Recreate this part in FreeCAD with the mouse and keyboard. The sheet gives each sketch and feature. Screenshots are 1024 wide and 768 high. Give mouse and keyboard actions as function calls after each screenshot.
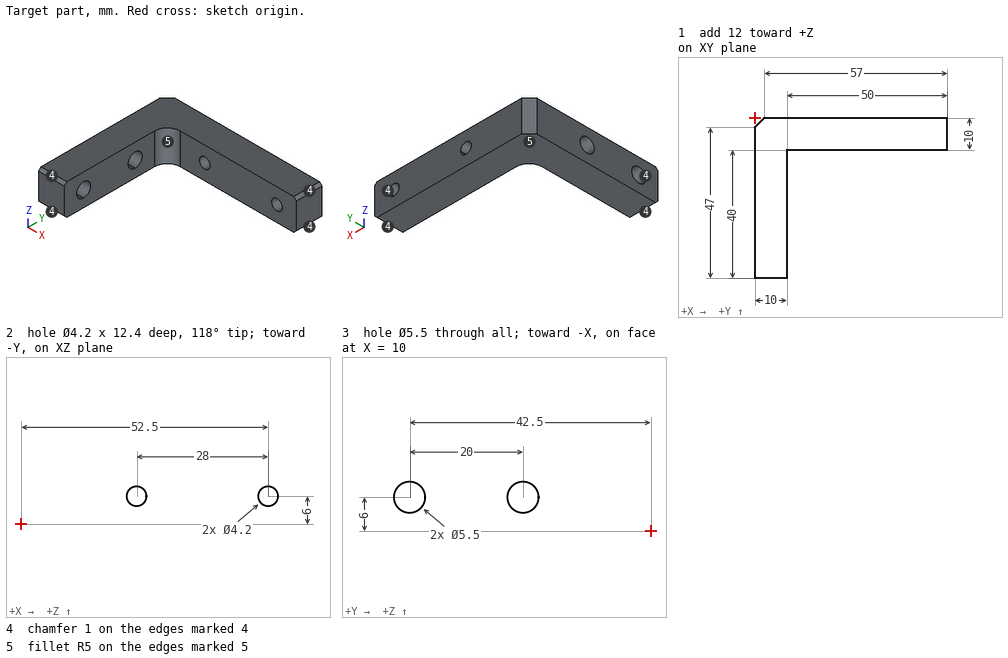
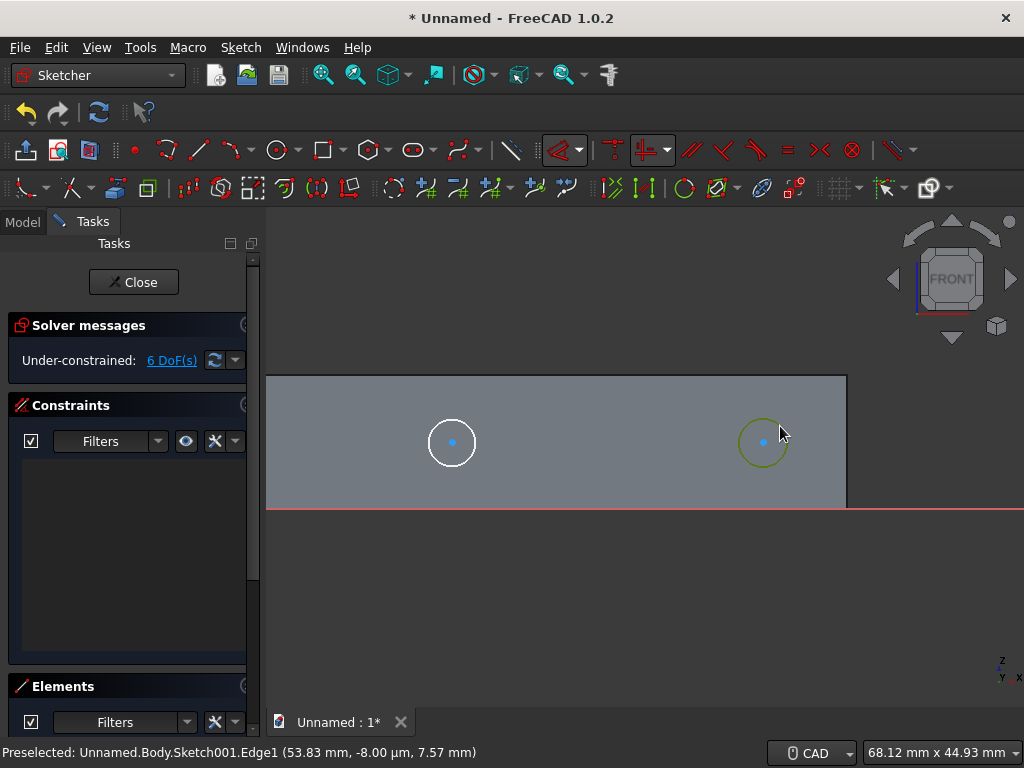
click(468, 426)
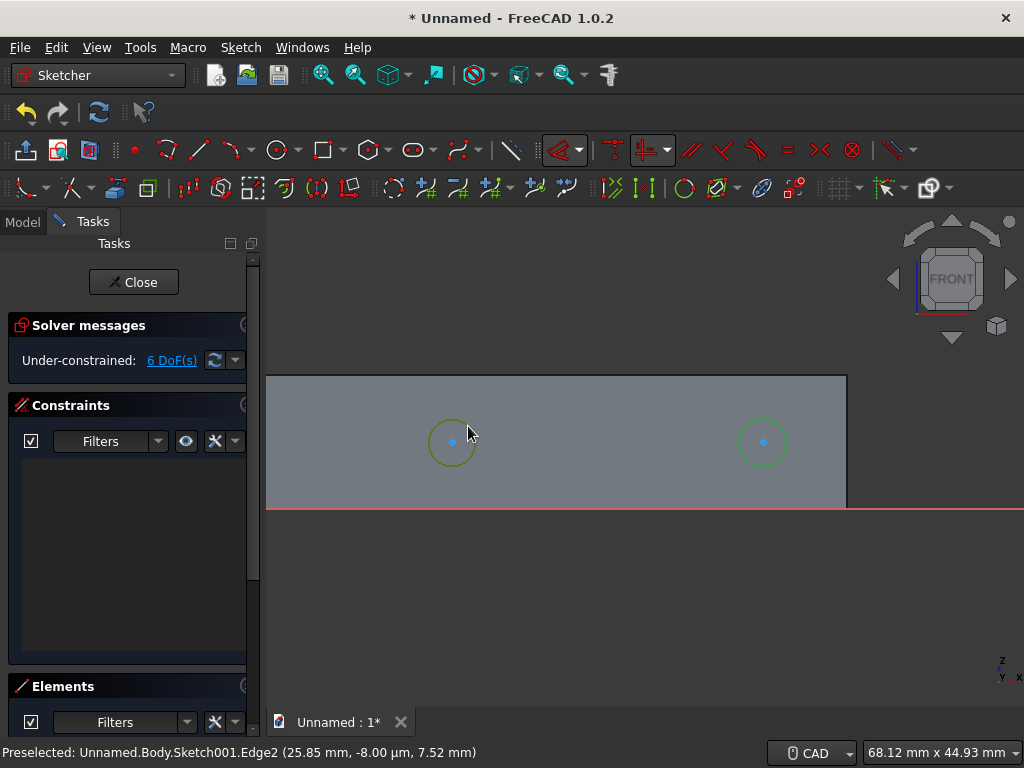
key(e)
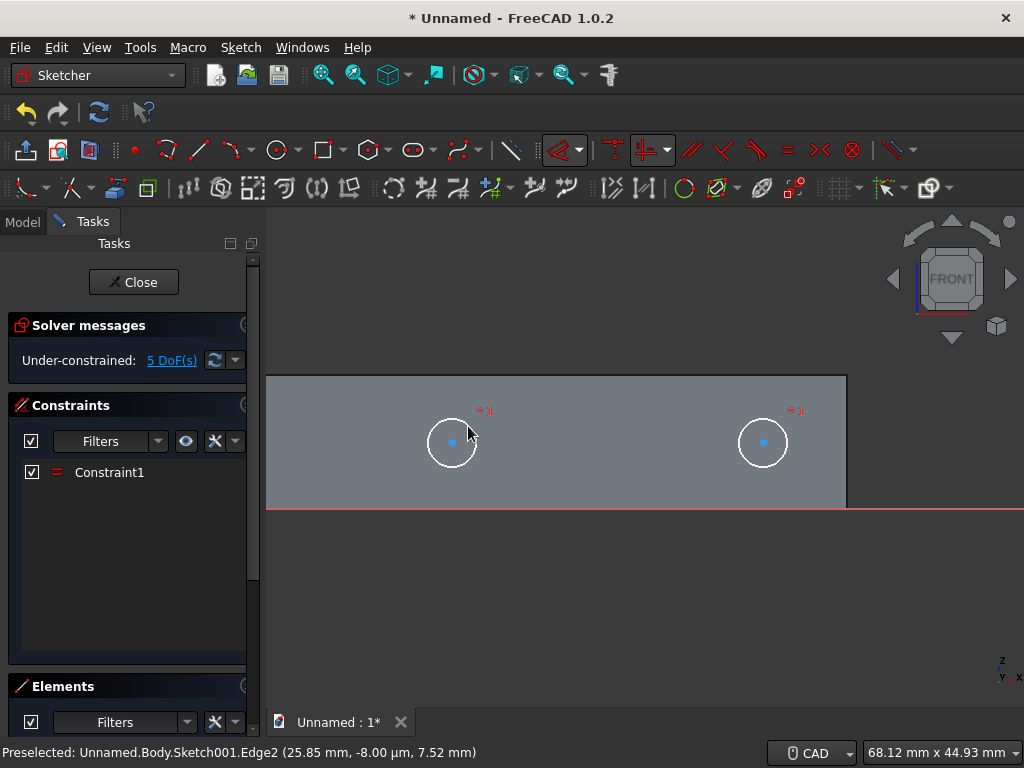
click(763, 443)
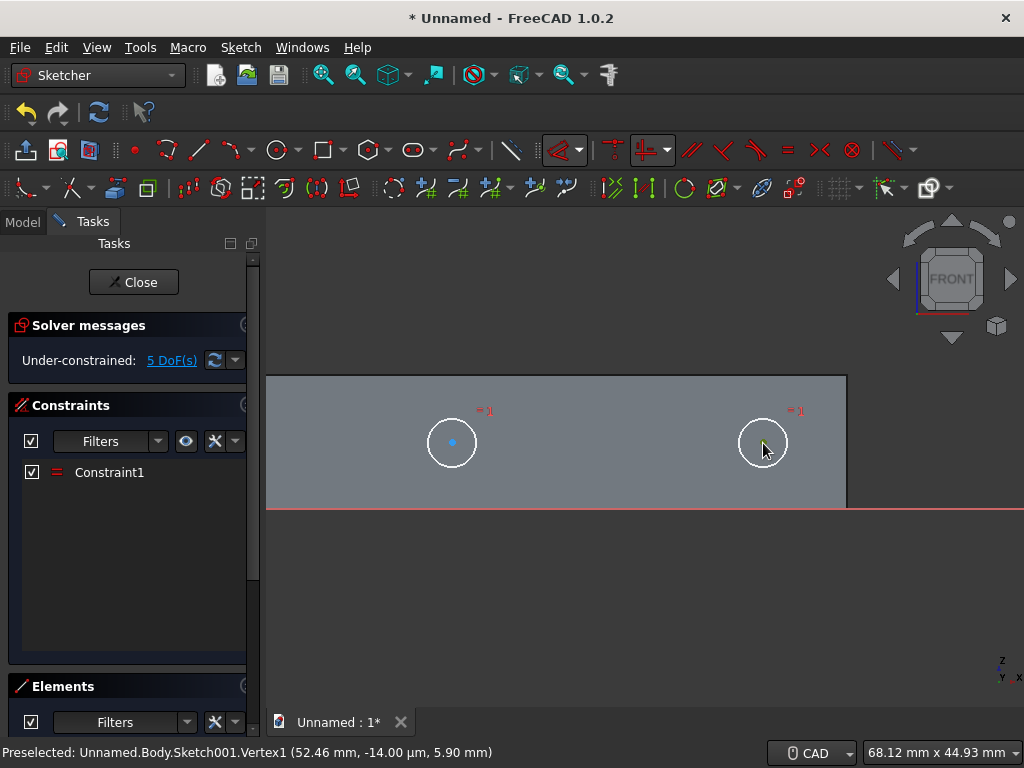
click(452, 443)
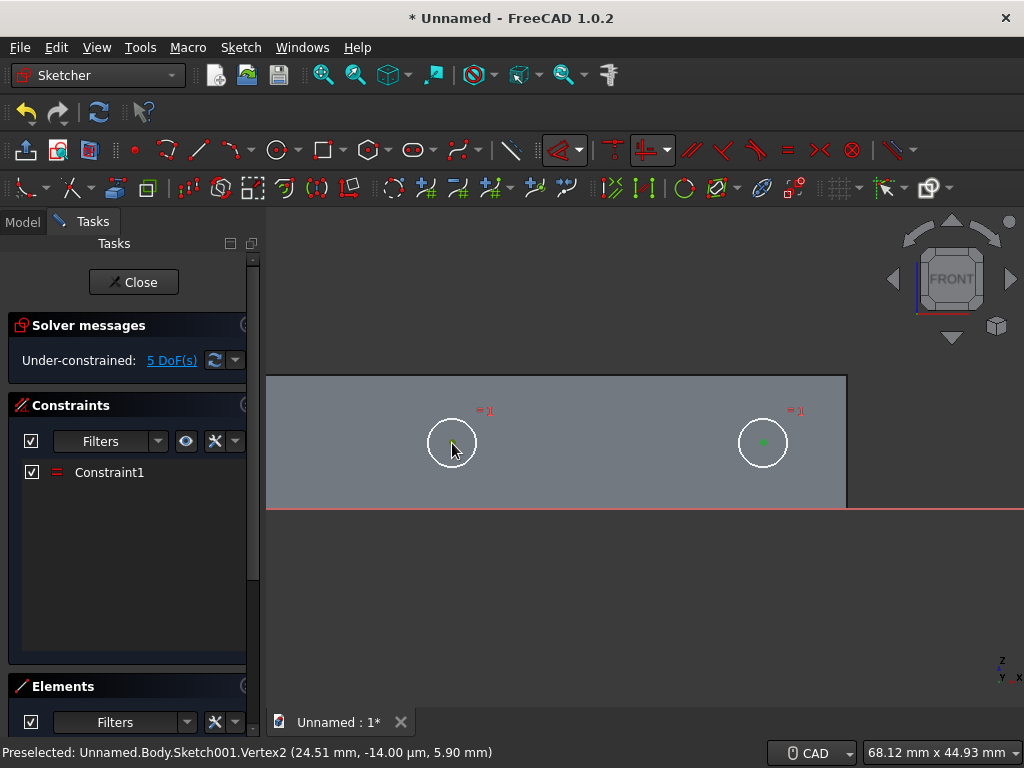
key(h)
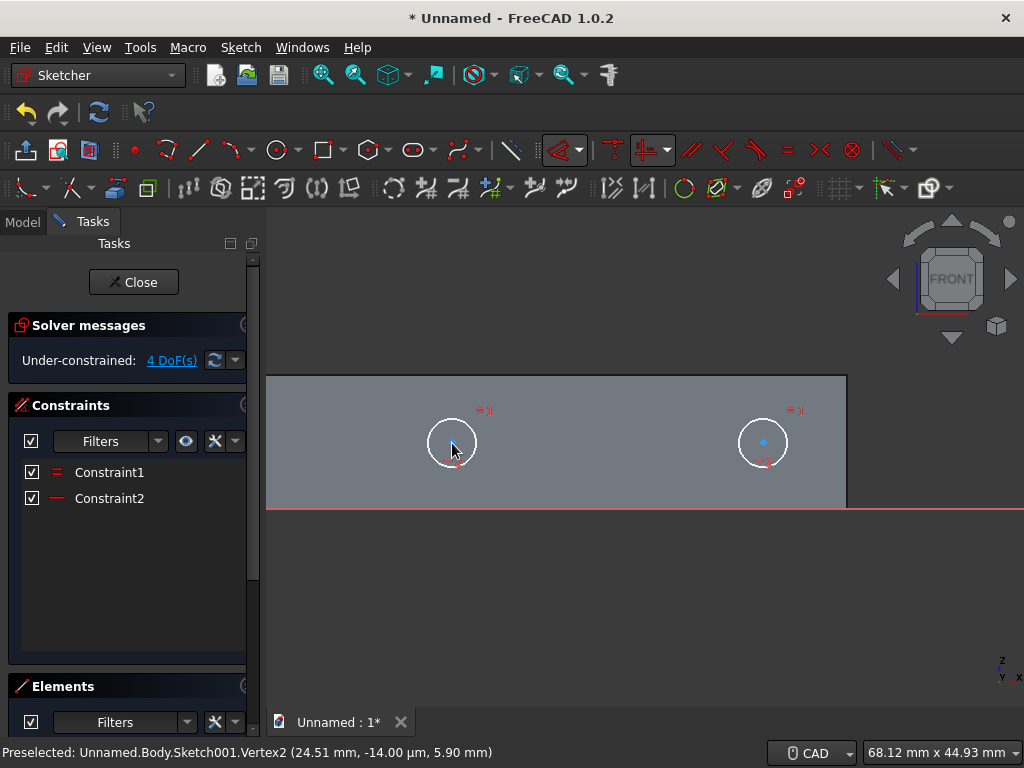
key(d)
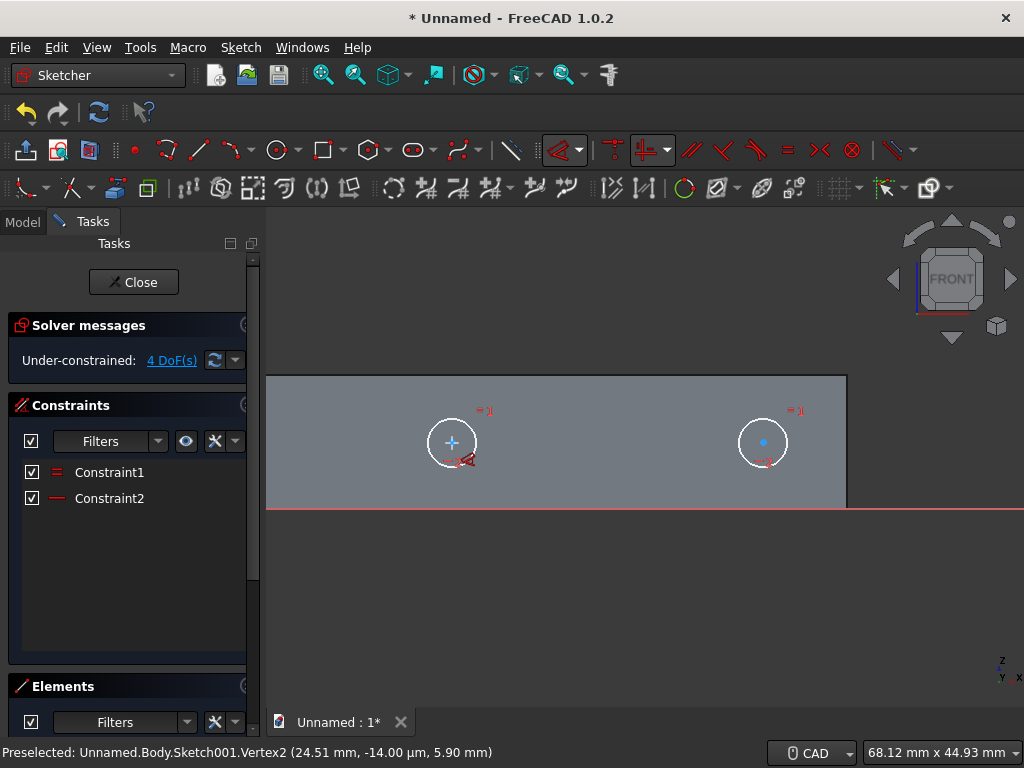
click(780, 426)
click(803, 403)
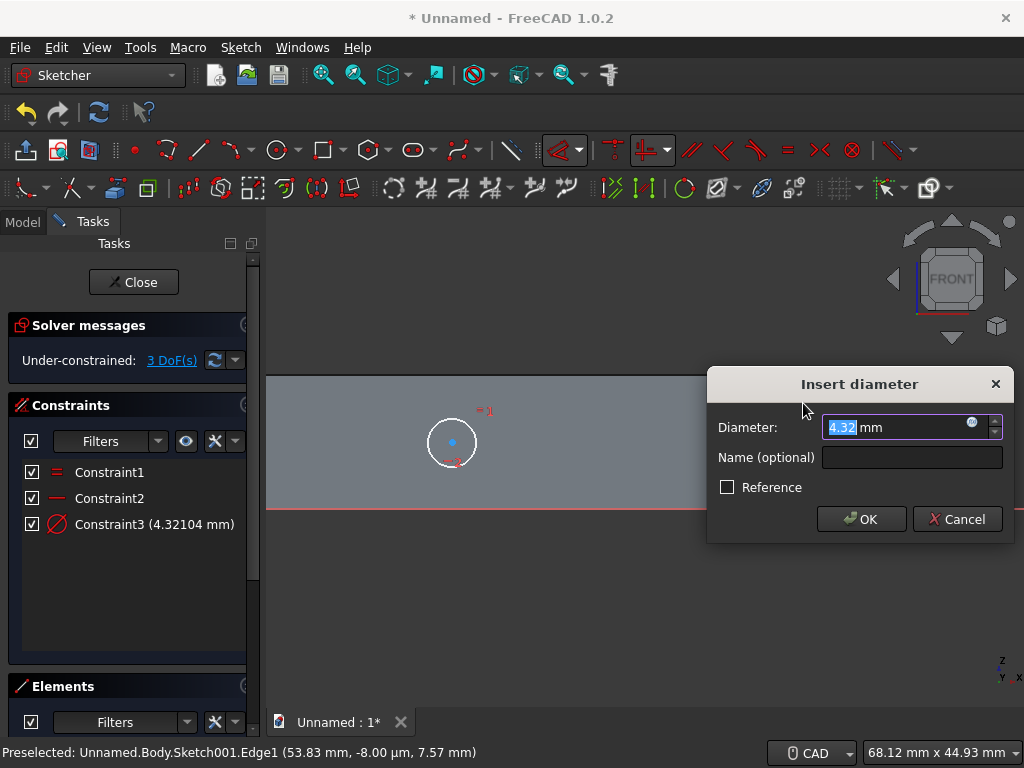
text(4.2)
key(Return)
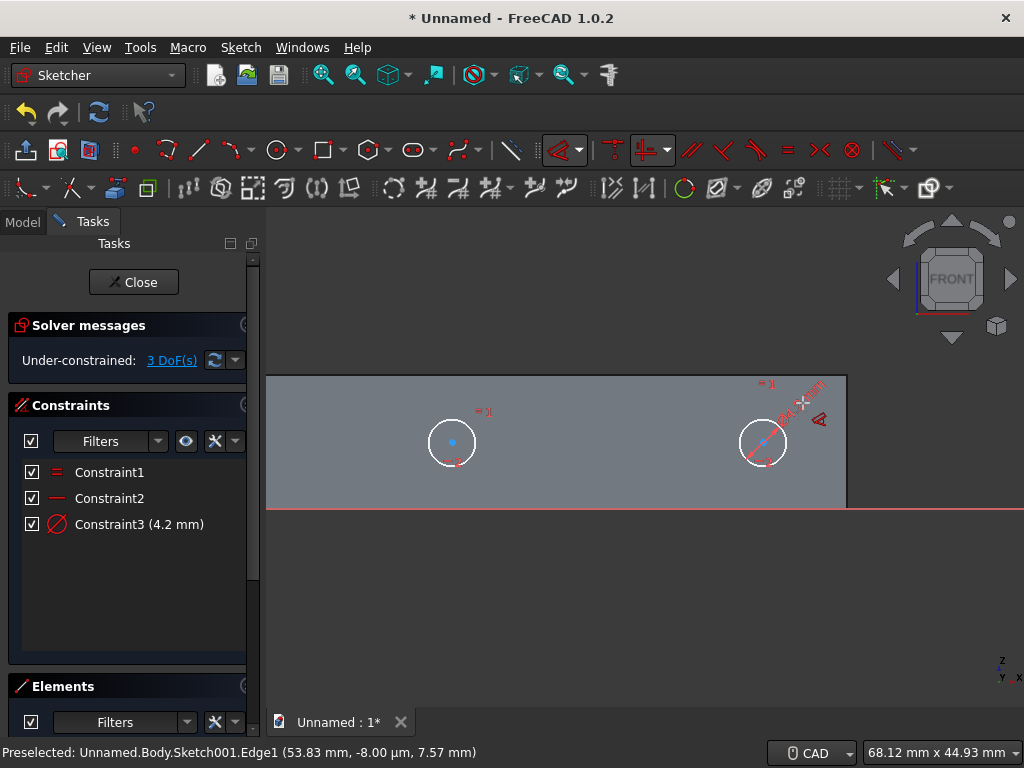
click(763, 443)
click(797, 476)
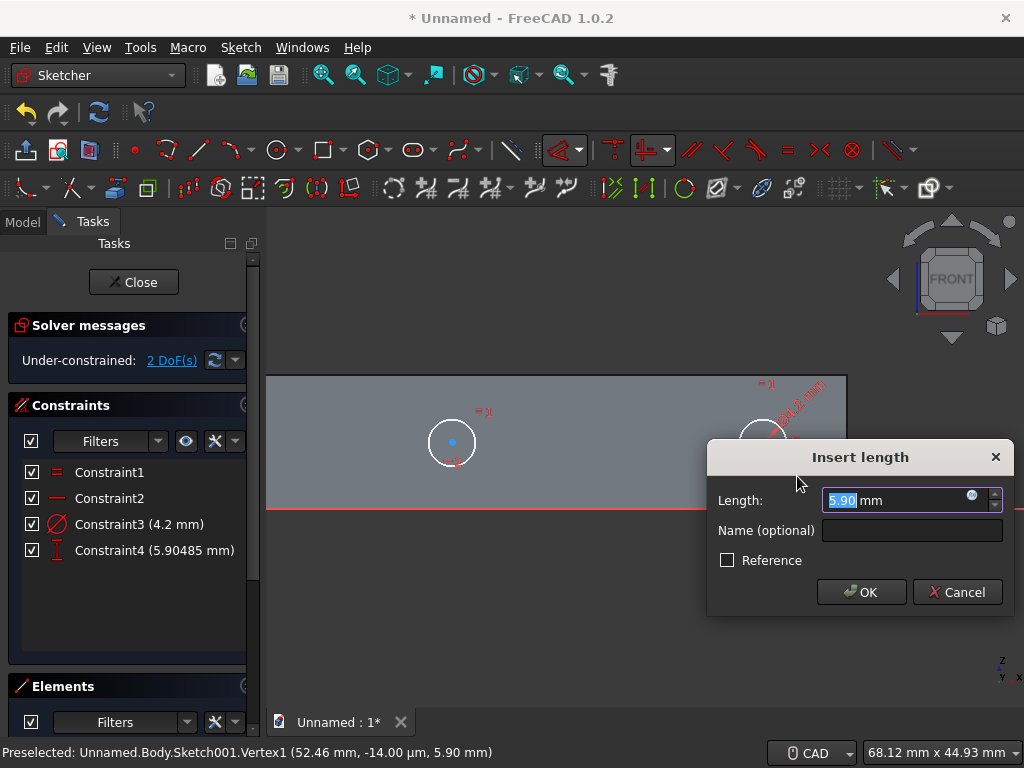
text(6)
key(Return)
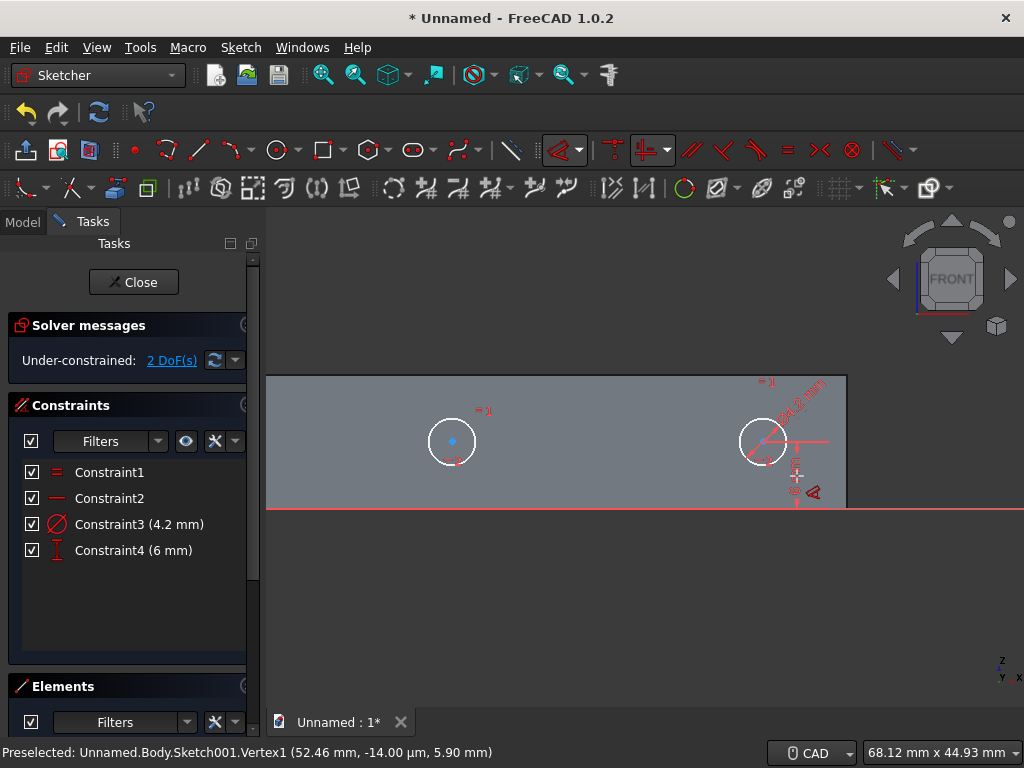
click(763, 442)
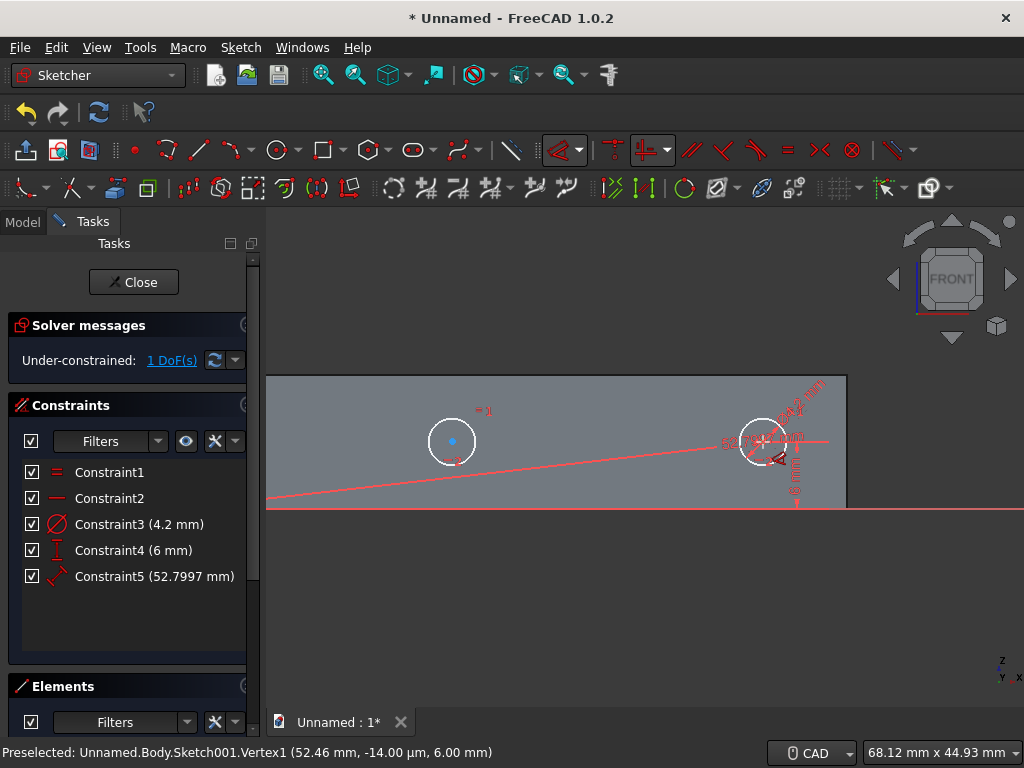
click(452, 442)
click(608, 408)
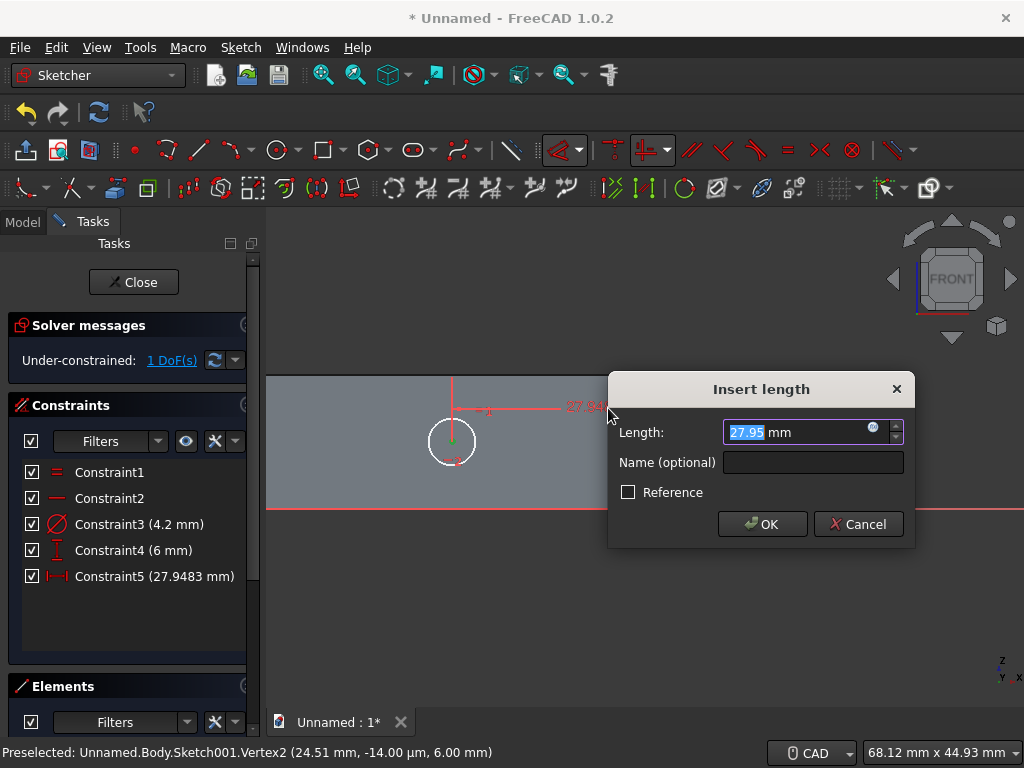
text(28)
key(Return)